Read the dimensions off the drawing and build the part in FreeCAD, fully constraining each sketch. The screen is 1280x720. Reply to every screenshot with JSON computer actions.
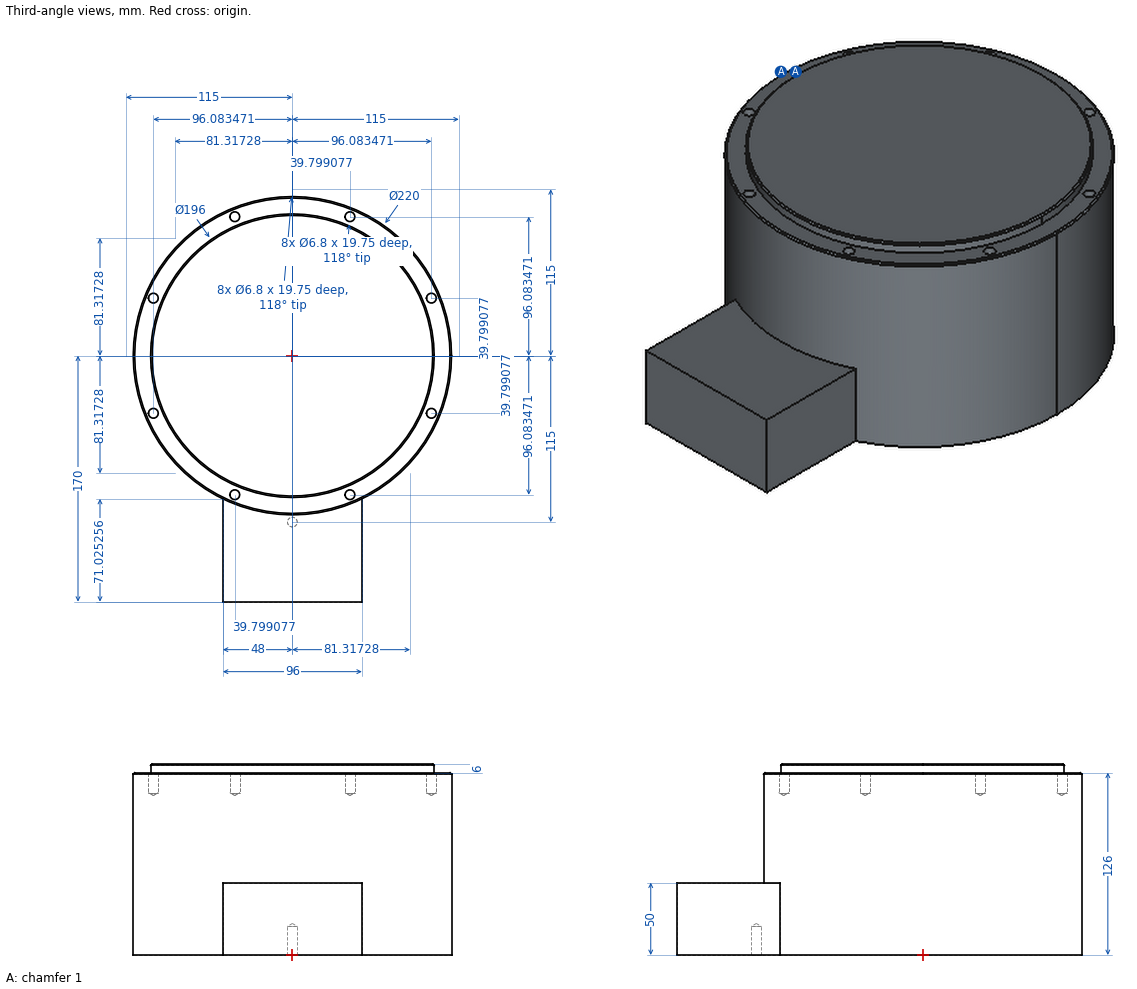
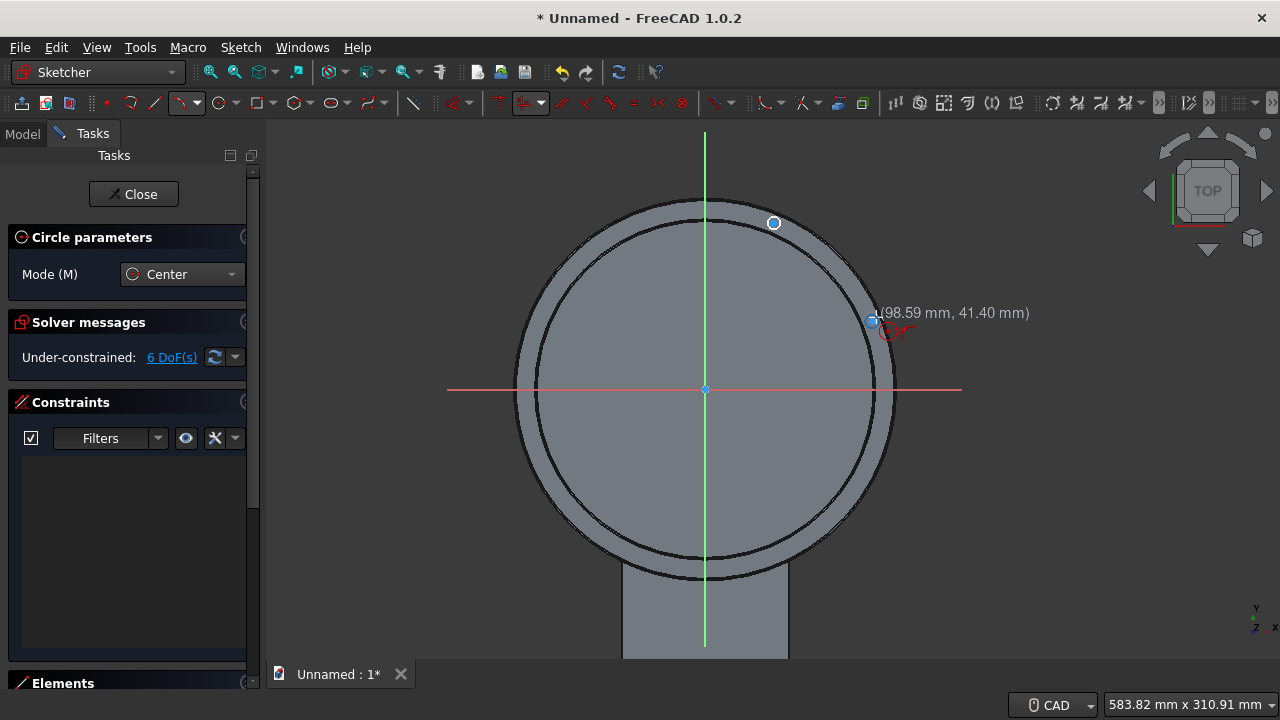
{"action": "scroll", "coordinate": [872, 459], "scroll_direction": "up", "scroll_amount": 7}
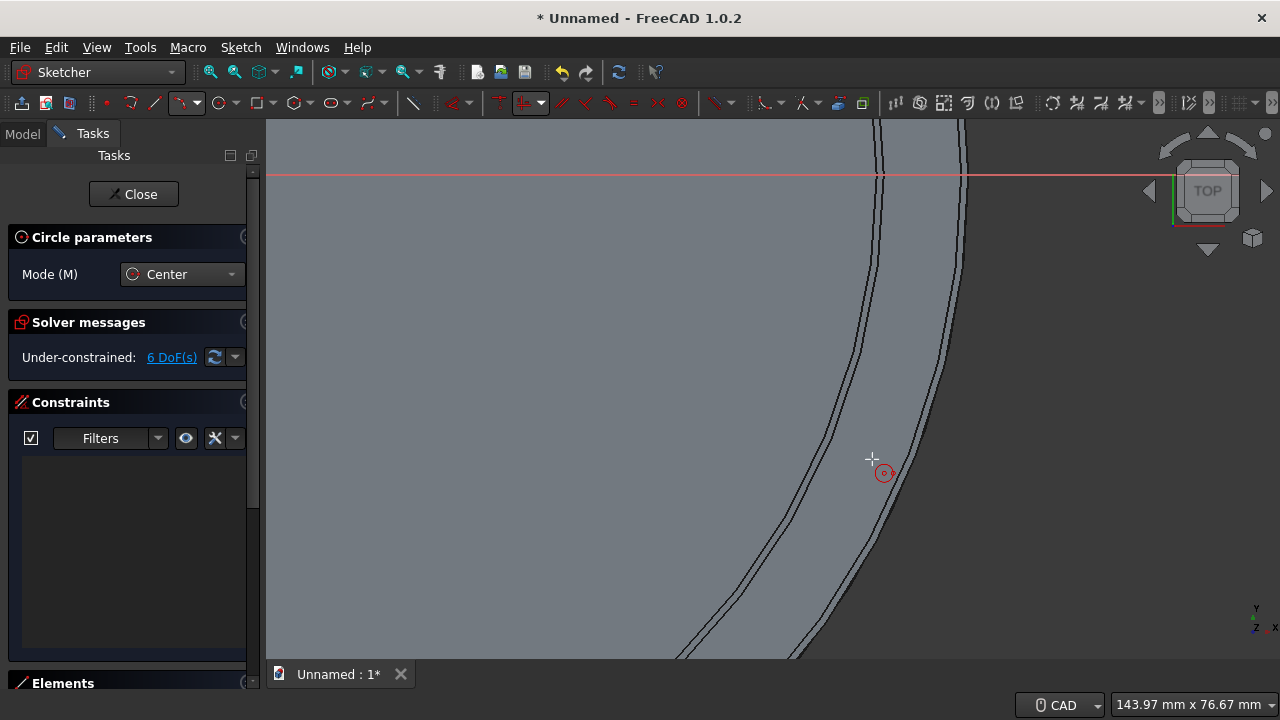
{"action": "scroll", "coordinate": [872, 459], "scroll_direction": "down", "scroll_amount": 7}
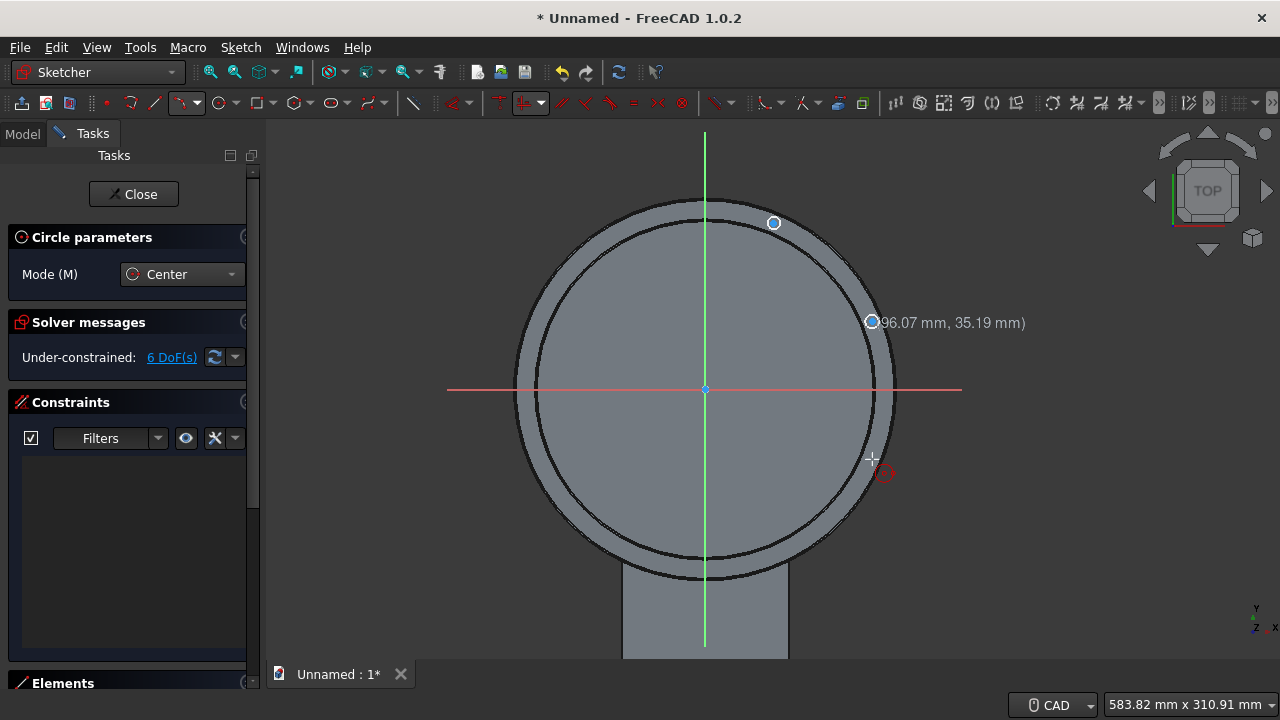
{"action": "left_click", "coordinate": [872, 459]}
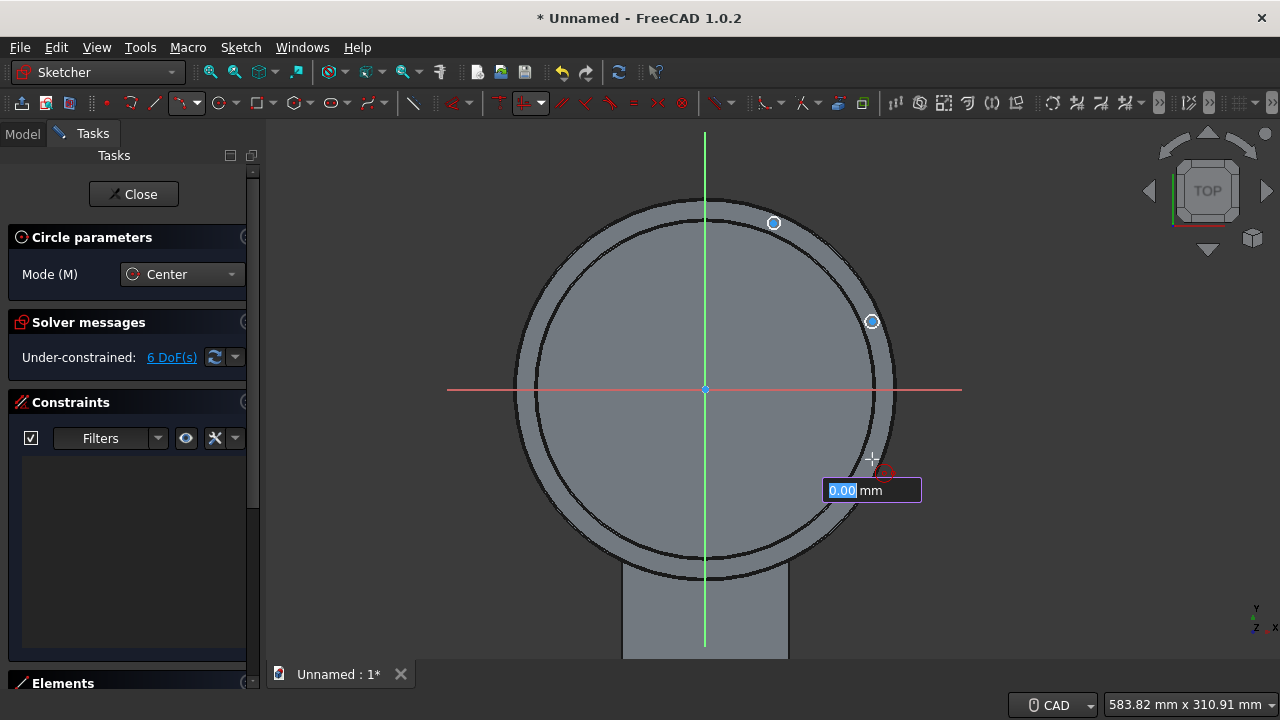
{"action": "scroll", "coordinate": [876, 454], "scroll_direction": "up", "scroll_amount": 5}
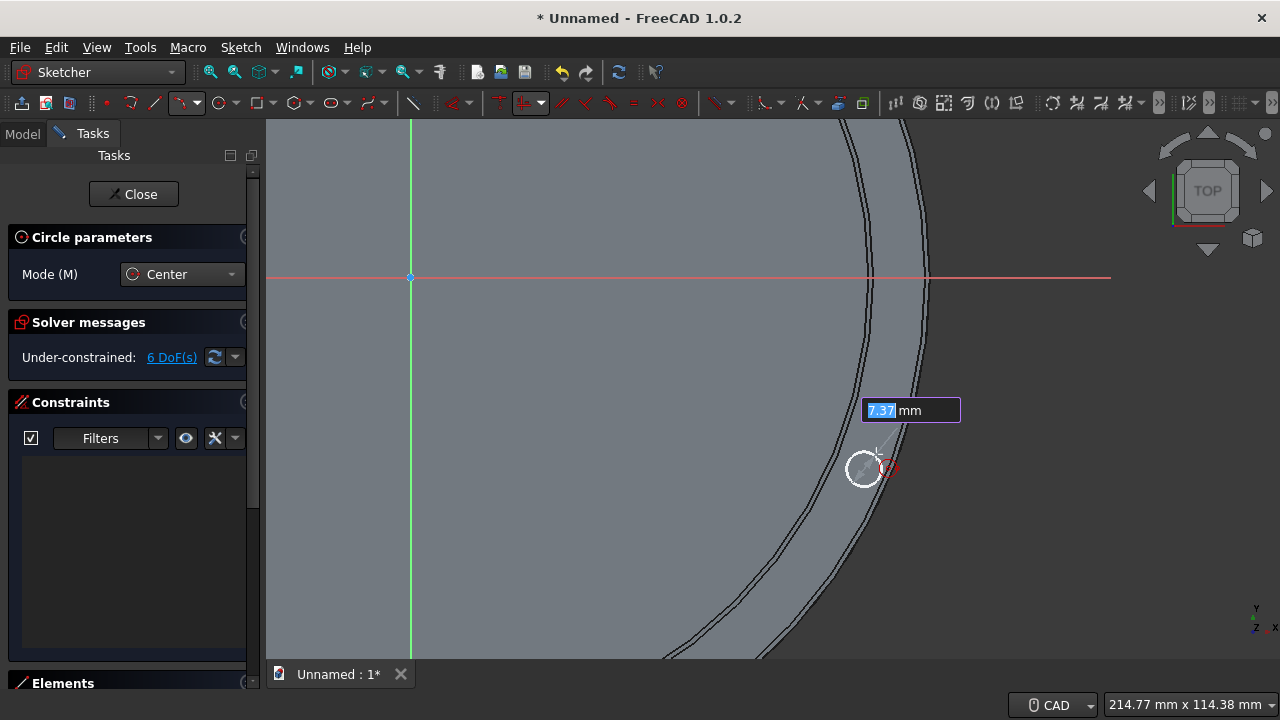
{"action": "left_click", "coordinate": [876, 454]}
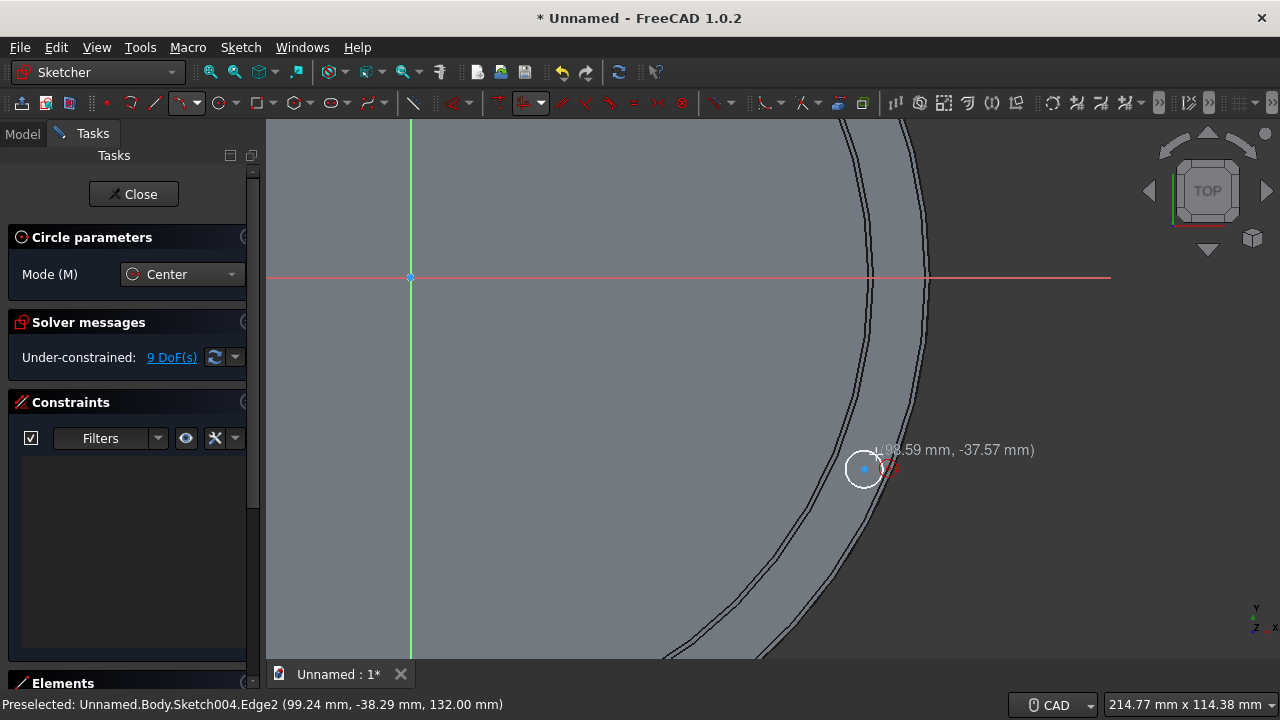
{"action": "scroll", "coordinate": [876, 454], "scroll_direction": "down", "scroll_amount": 5}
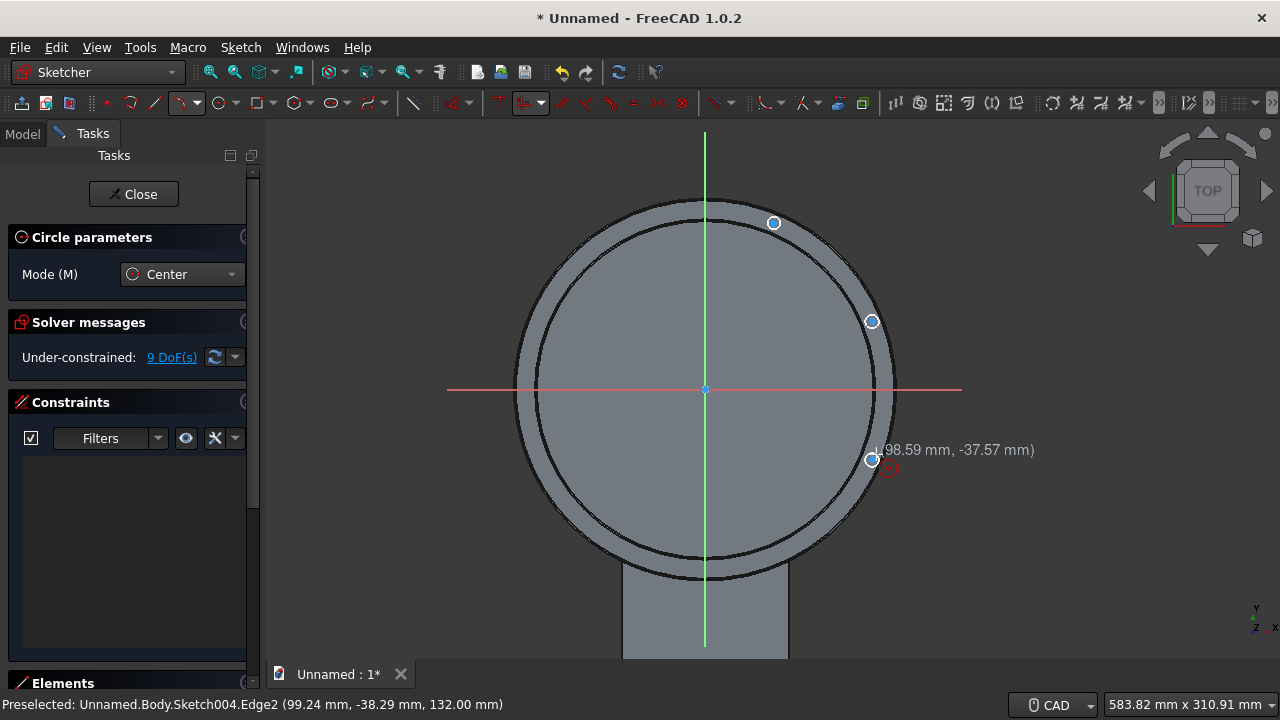
{"action": "scroll", "coordinate": [774, 556], "scroll_direction": "up", "scroll_amount": 7}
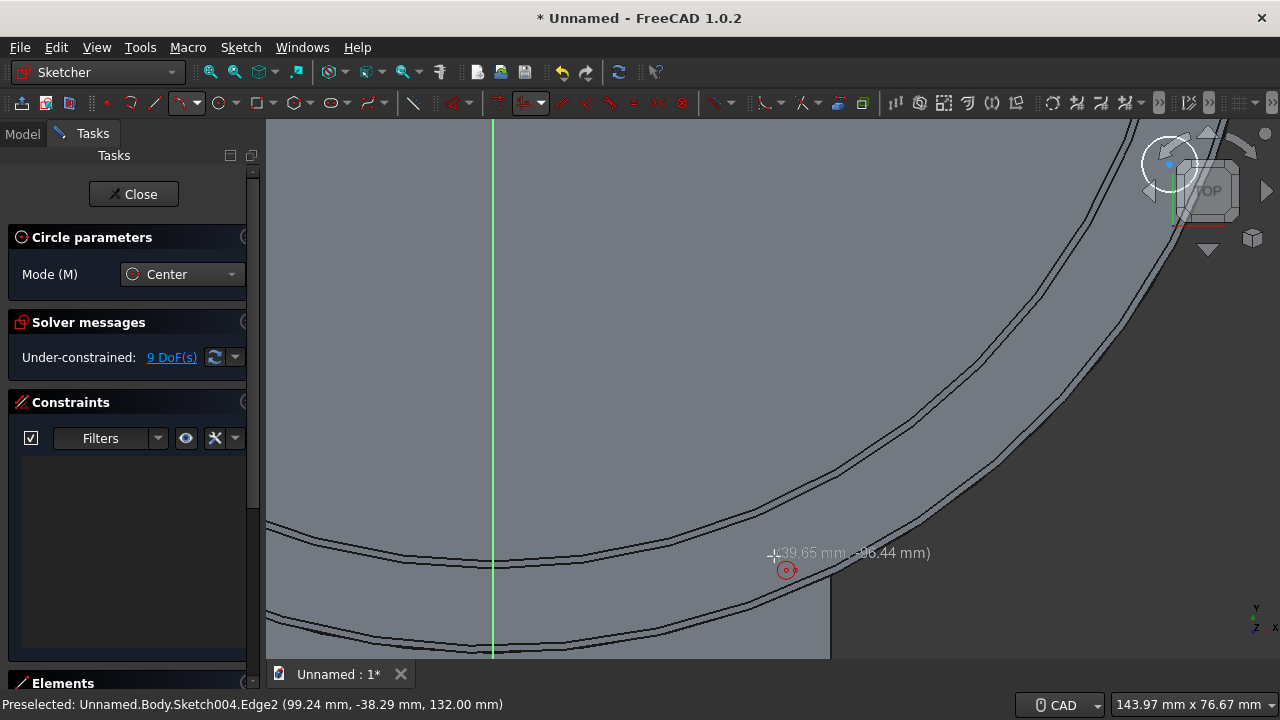
{"action": "scroll", "coordinate": [774, 556], "scroll_direction": "down", "scroll_amount": 7}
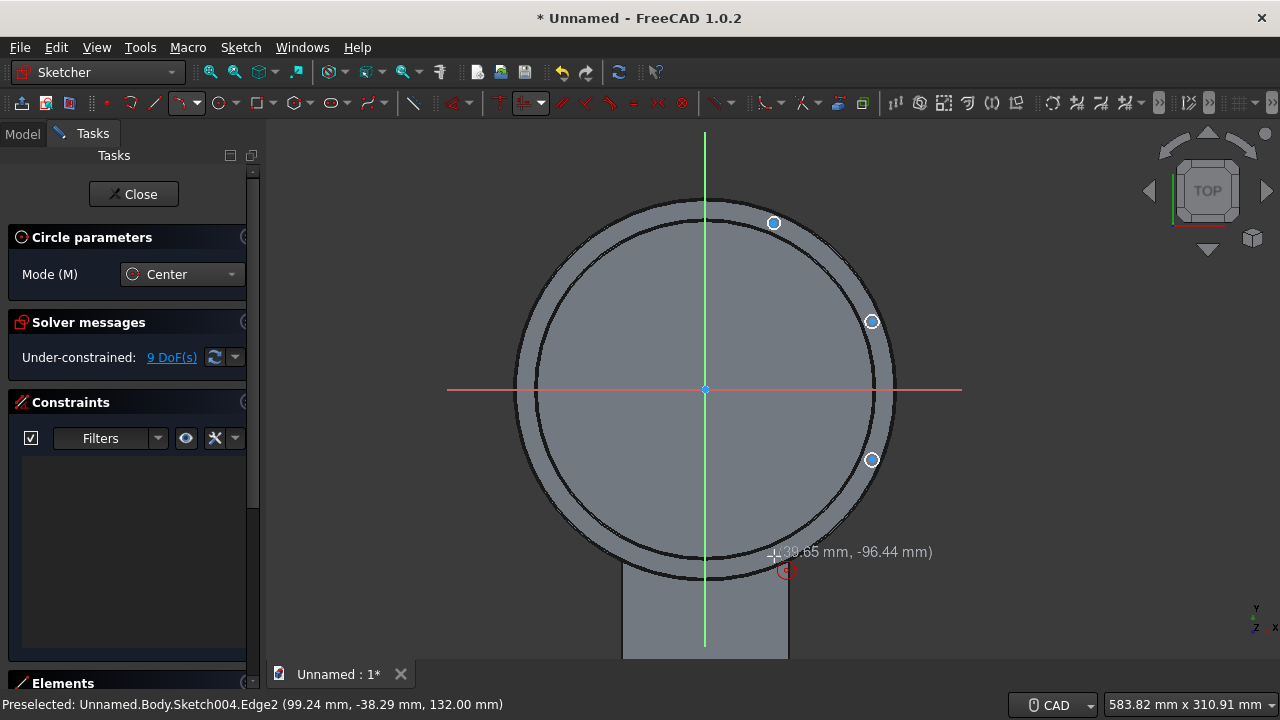
{"action": "left_click", "coordinate": [774, 556]}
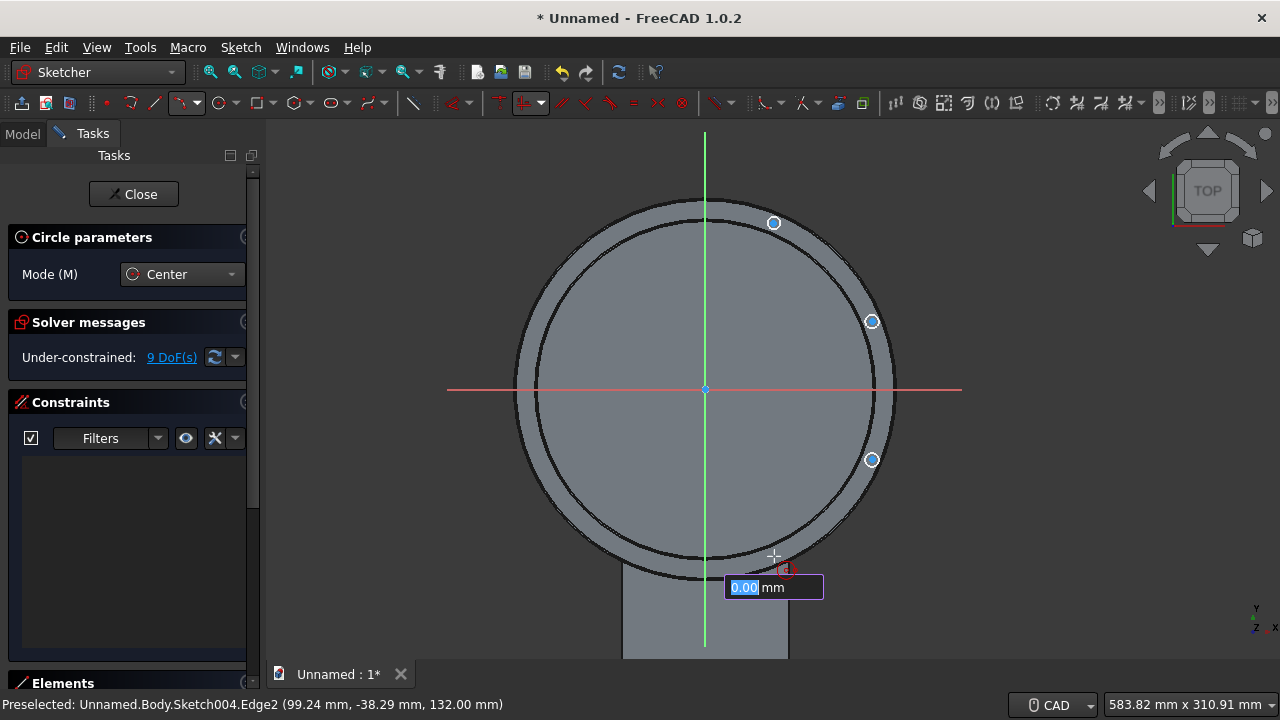
{"action": "scroll", "coordinate": [778, 552], "scroll_direction": "up", "scroll_amount": 5}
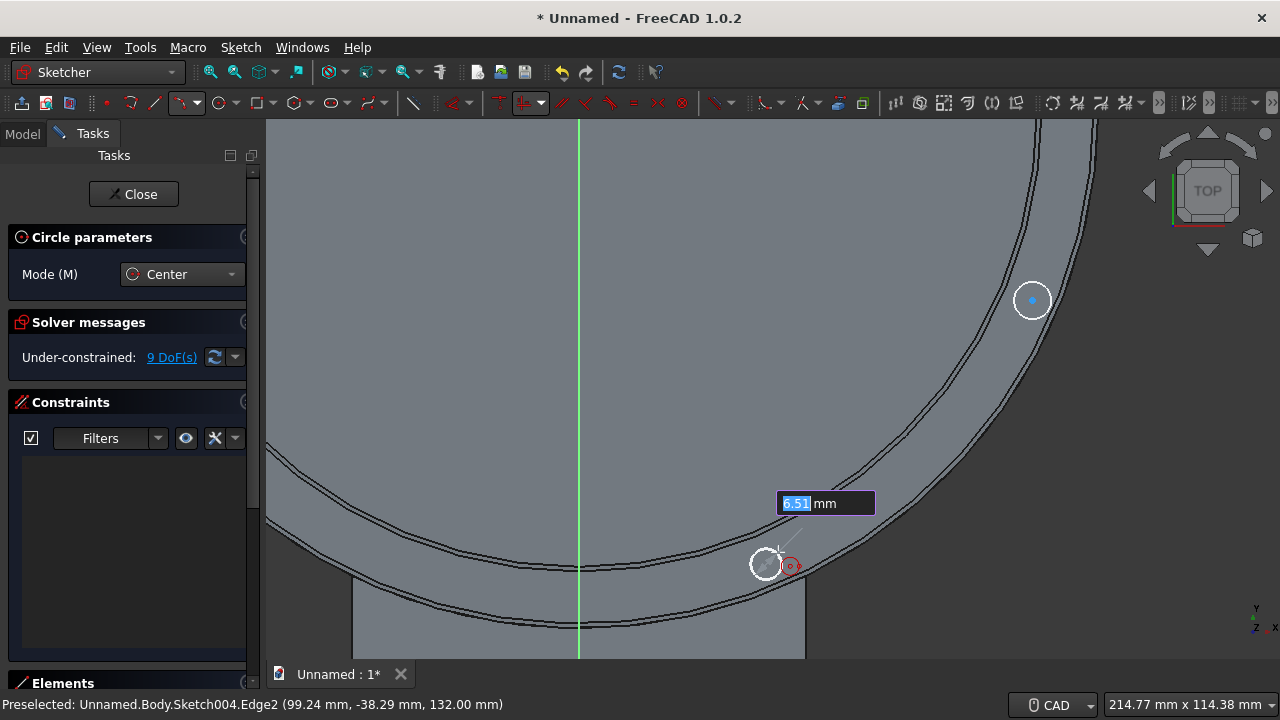
{"action": "left_click", "coordinate": [778, 551]}